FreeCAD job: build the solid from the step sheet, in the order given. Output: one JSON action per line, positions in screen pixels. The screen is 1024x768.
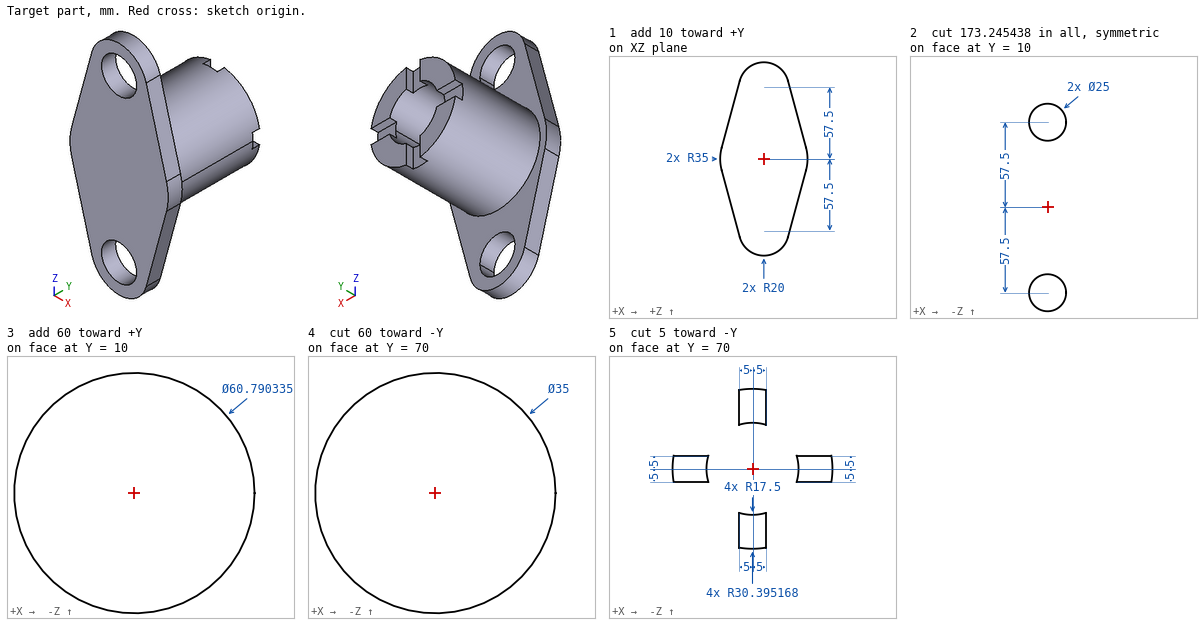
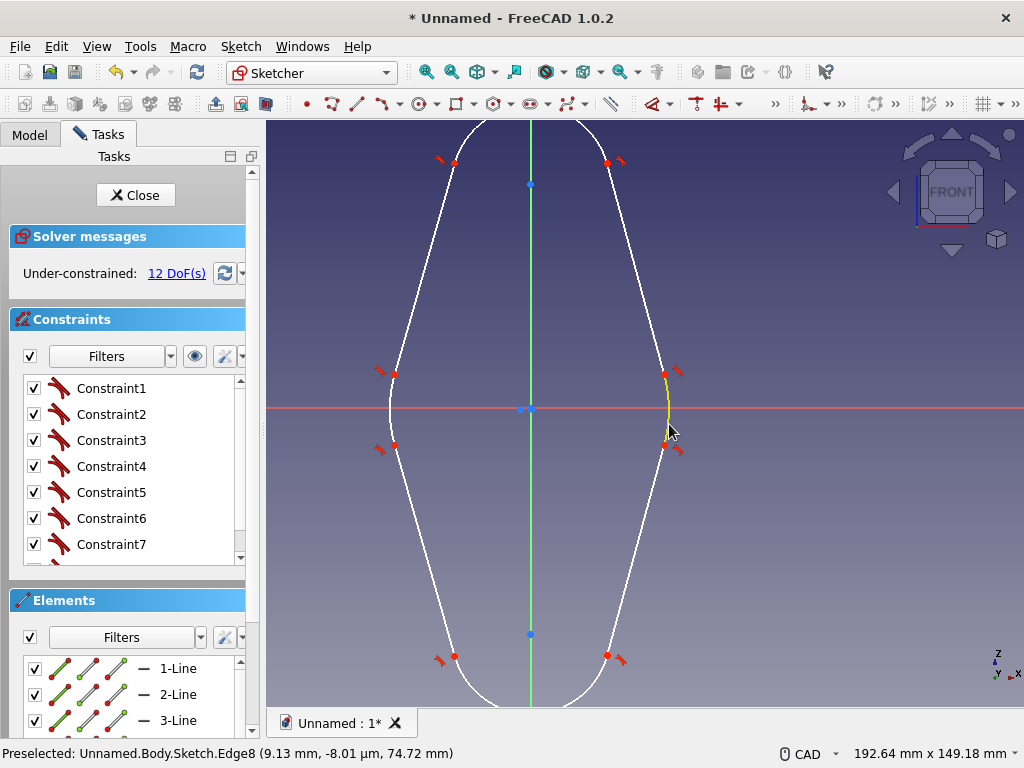
{"action": "left_click", "coordinate": [668, 424]}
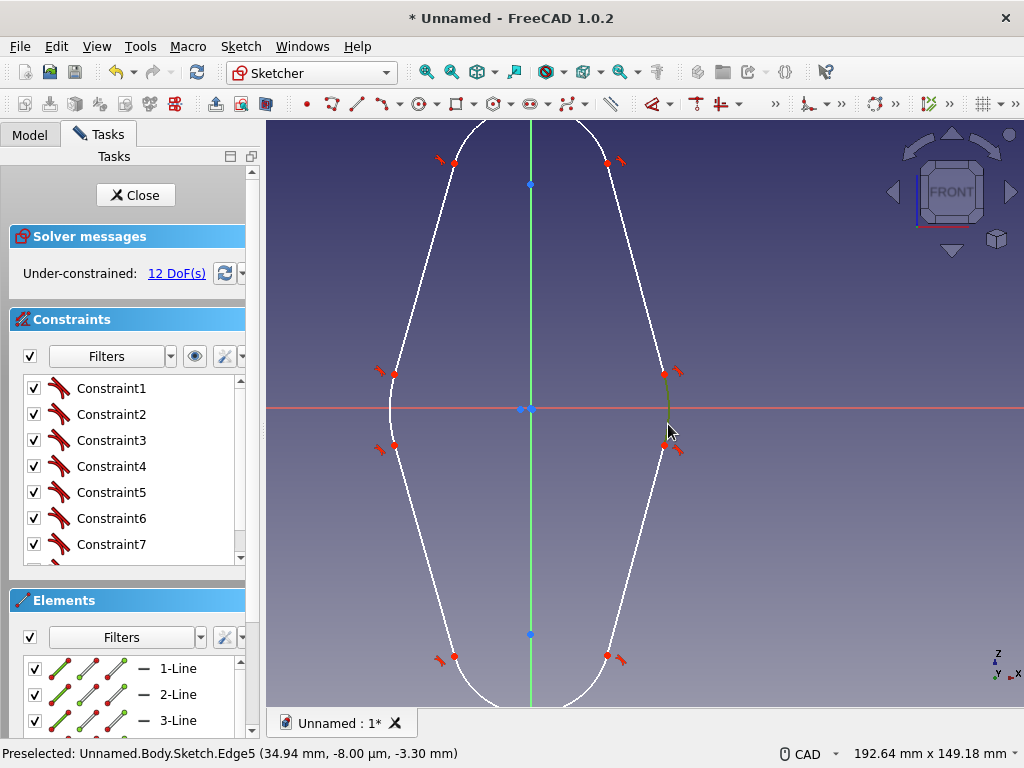
{"action": "left_click", "coordinate": [391, 395]}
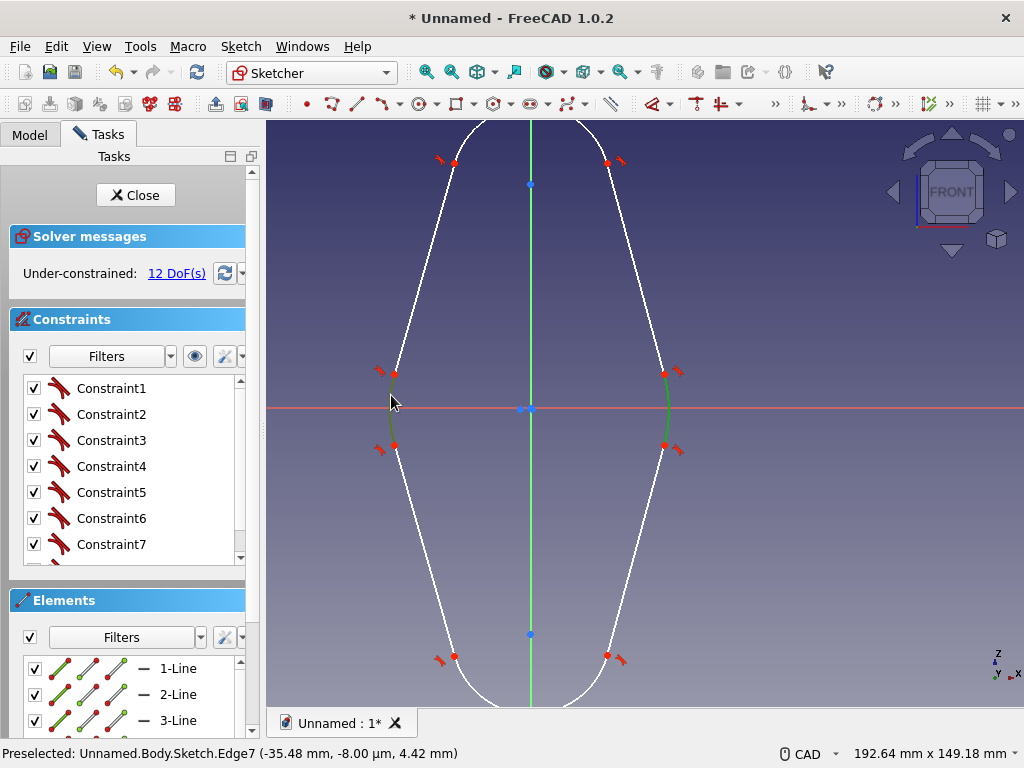
{"action": "left_click", "coordinate": [696, 104]}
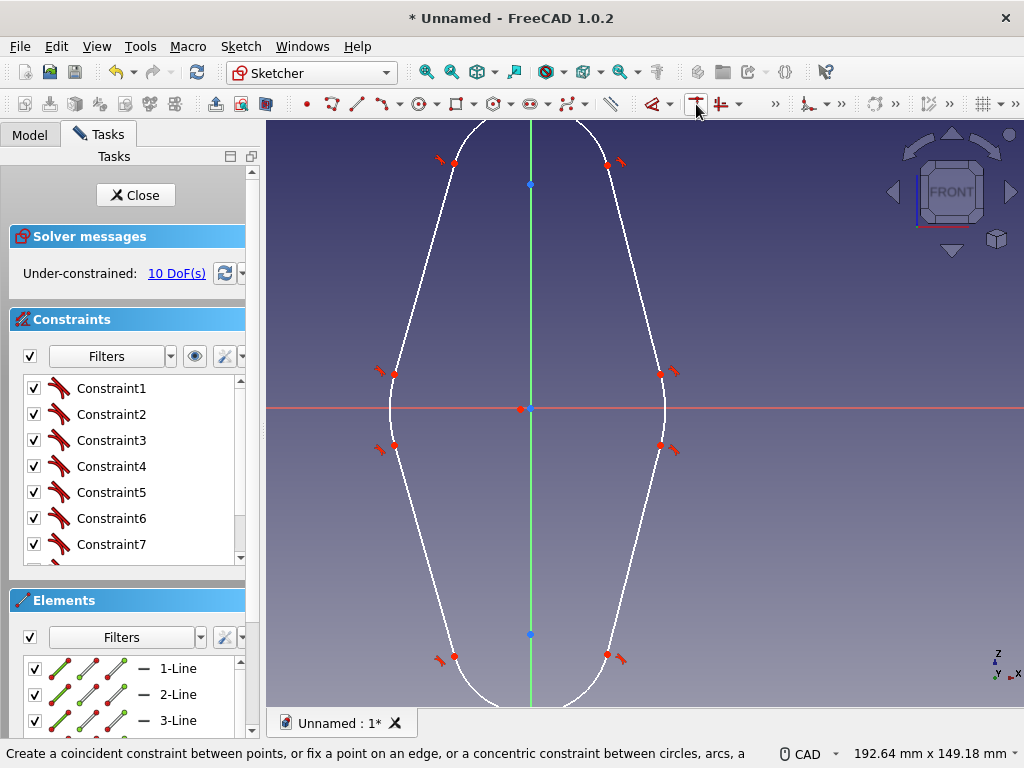
{"action": "left_click_drag", "start_coordinate": [511, 398], "coordinate": [541, 420]}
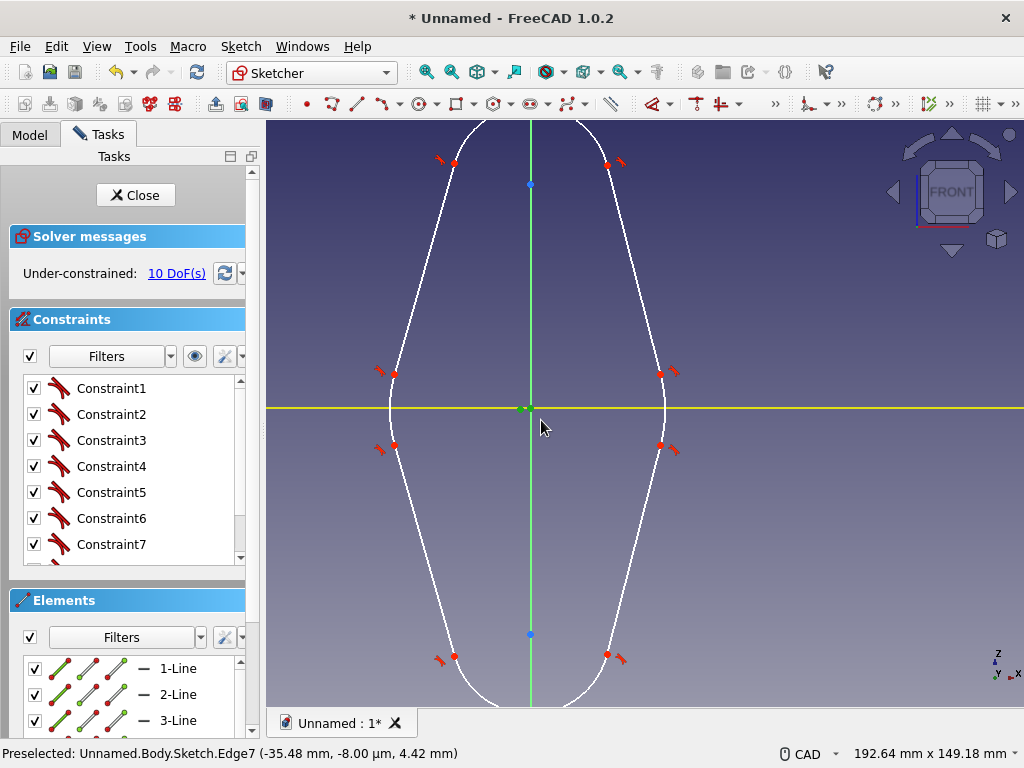
{"action": "left_click", "coordinate": [696, 104]}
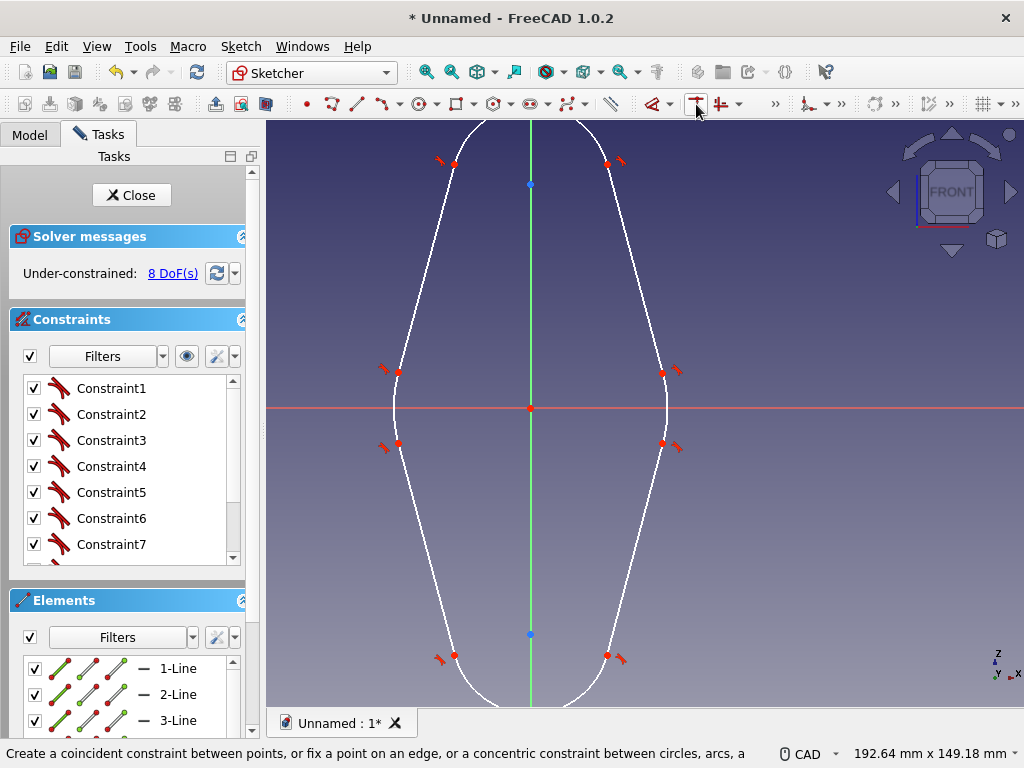
{"action": "left_click", "coordinate": [667, 422]}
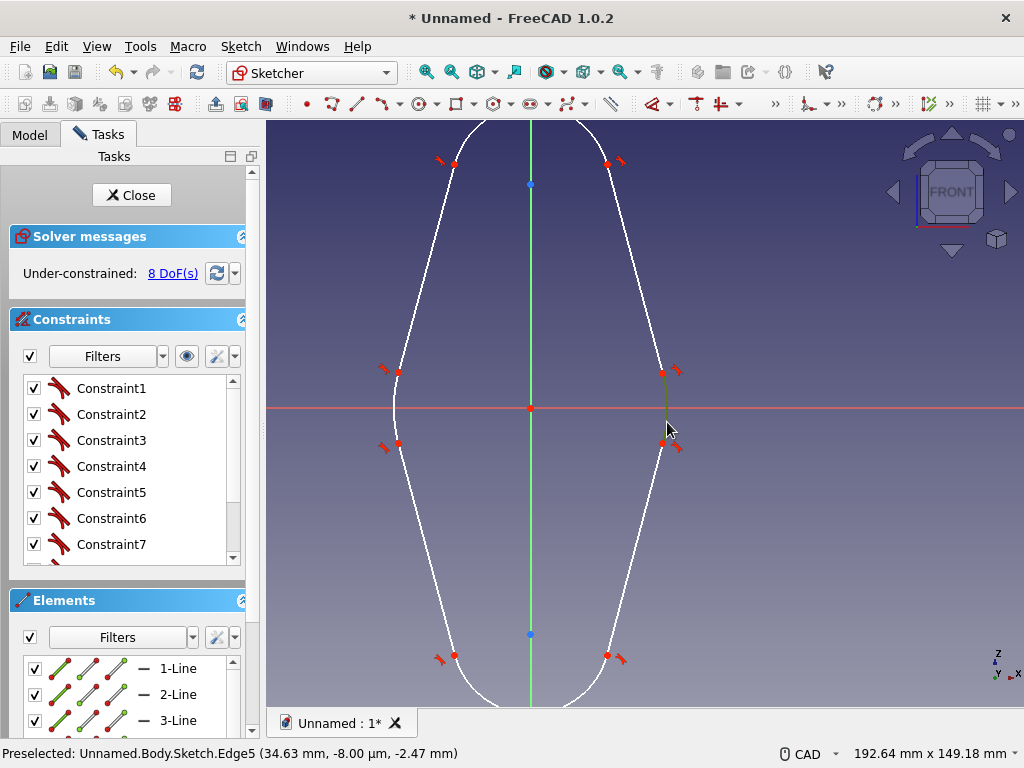
{"action": "left_click", "coordinate": [395, 394]}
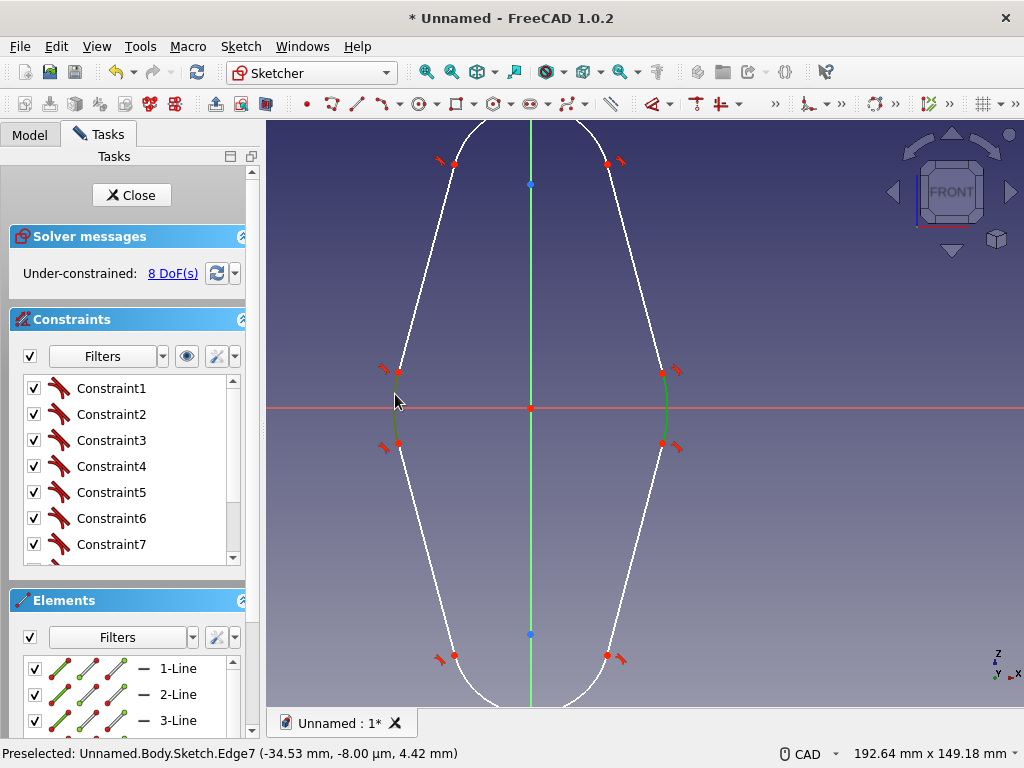
{"action": "key", "text": "e"}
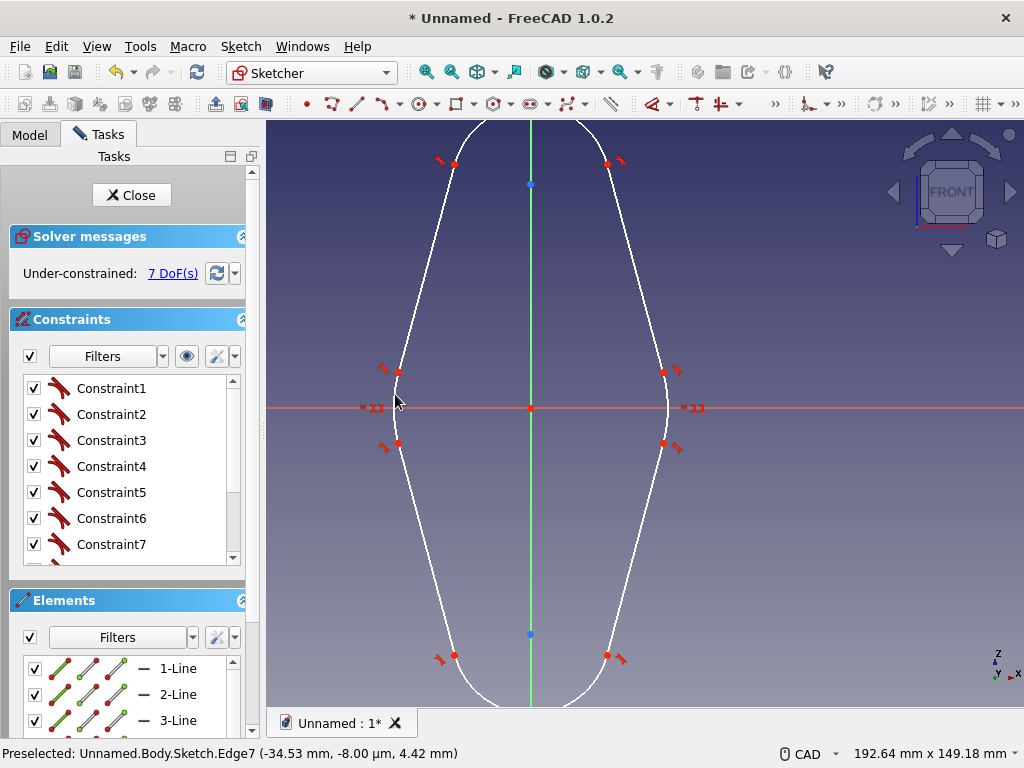
{"action": "scroll", "coordinate": [669, 424], "scroll_direction": "down", "scroll_amount": 2}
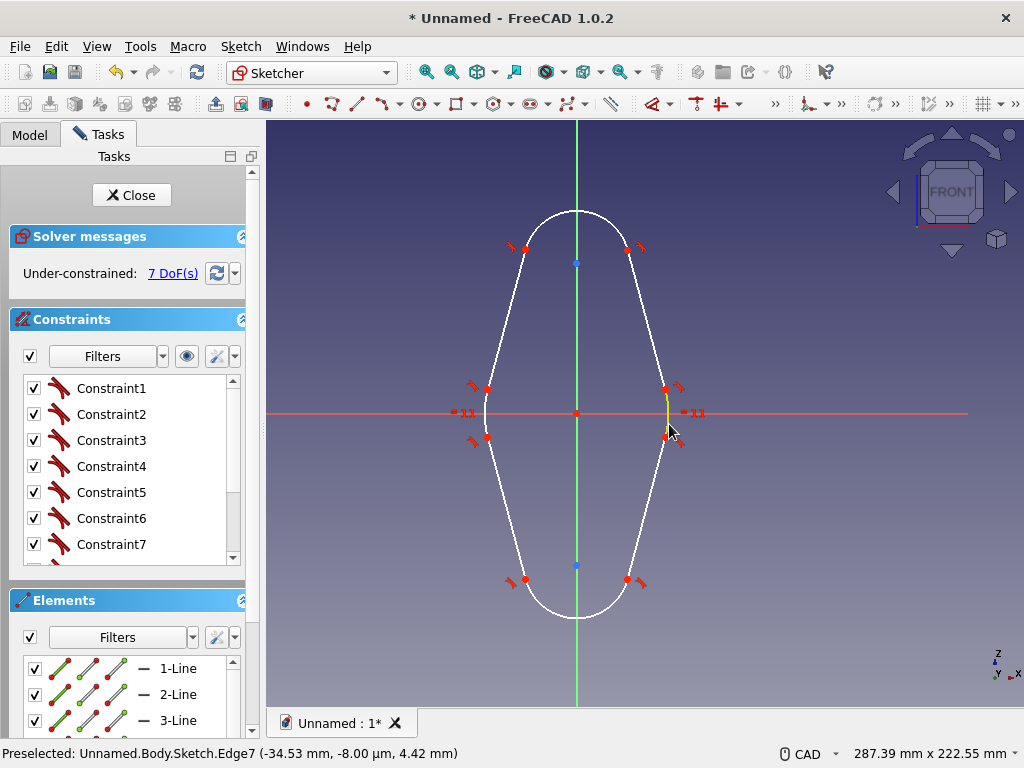
{"action": "left_click", "coordinate": [550, 611]}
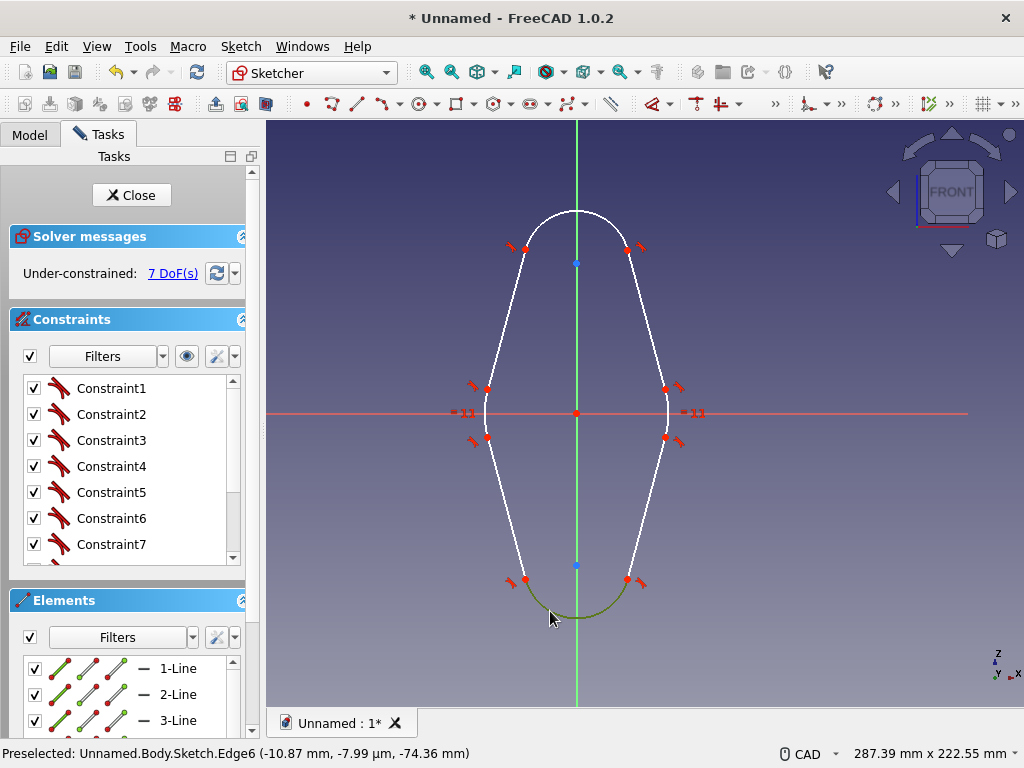
{"action": "left_click", "coordinate": [603, 218]}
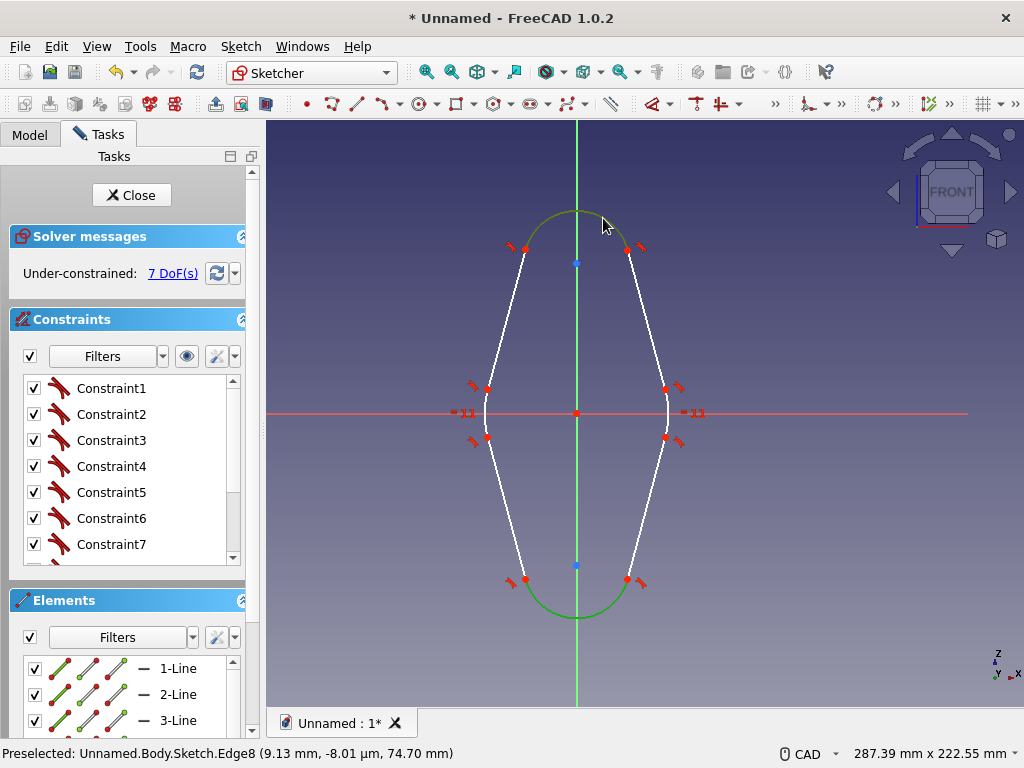
{"action": "key", "text": "e"}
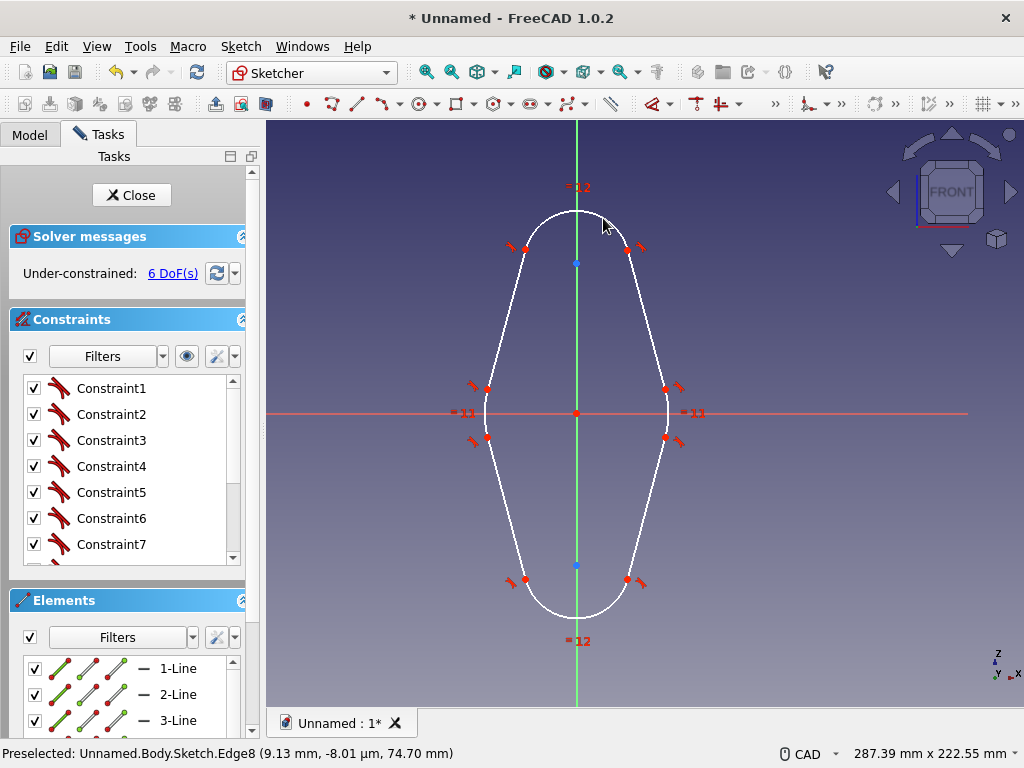
{"action": "left_click", "coordinate": [577, 566]}